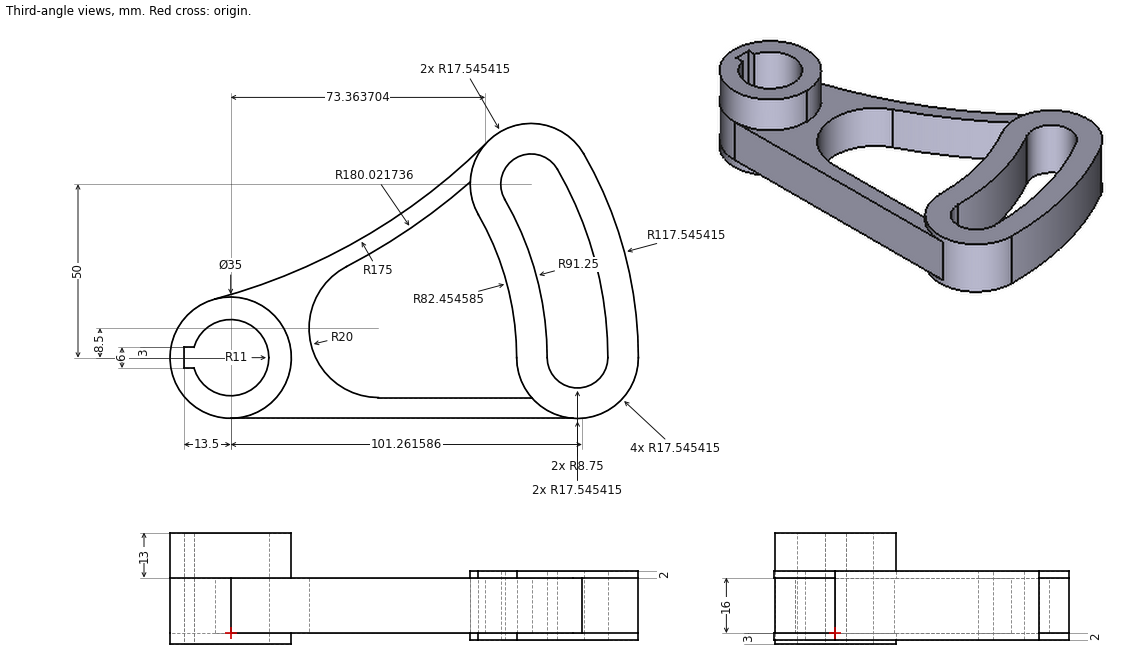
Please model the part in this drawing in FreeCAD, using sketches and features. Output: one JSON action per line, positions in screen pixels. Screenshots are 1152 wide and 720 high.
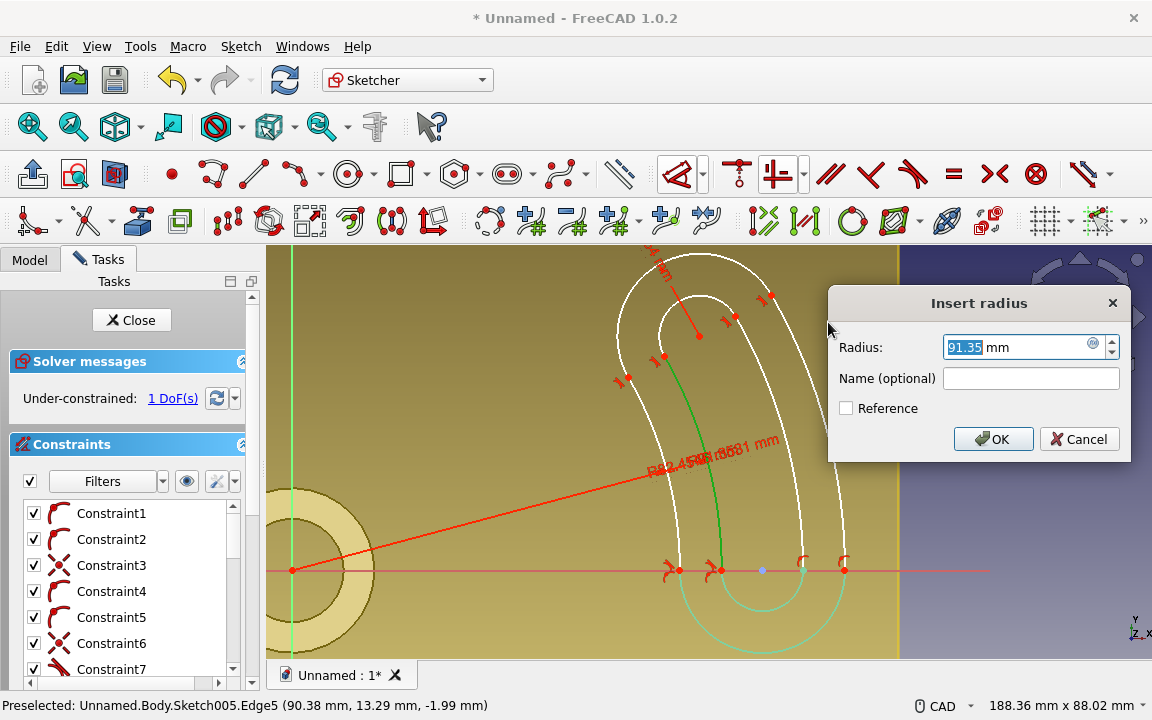
{"action": "type", "text": "91.25"}
{"action": "key", "text": "Return"}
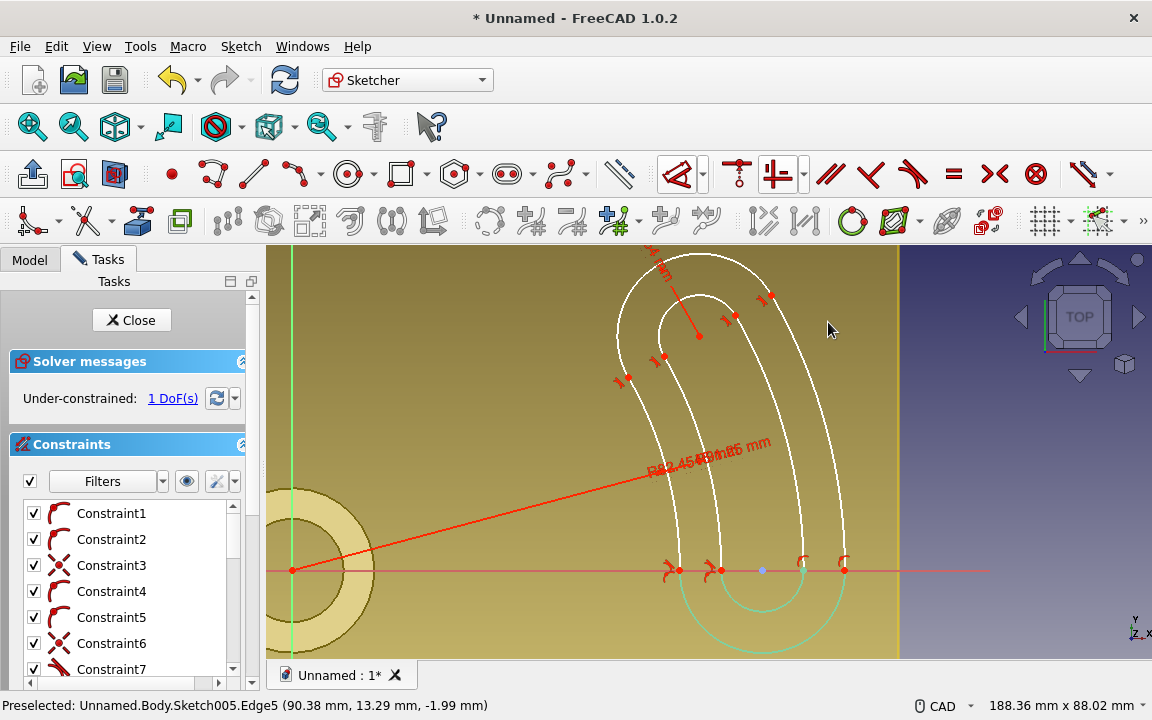
{"action": "left_click", "coordinate": [700, 336]}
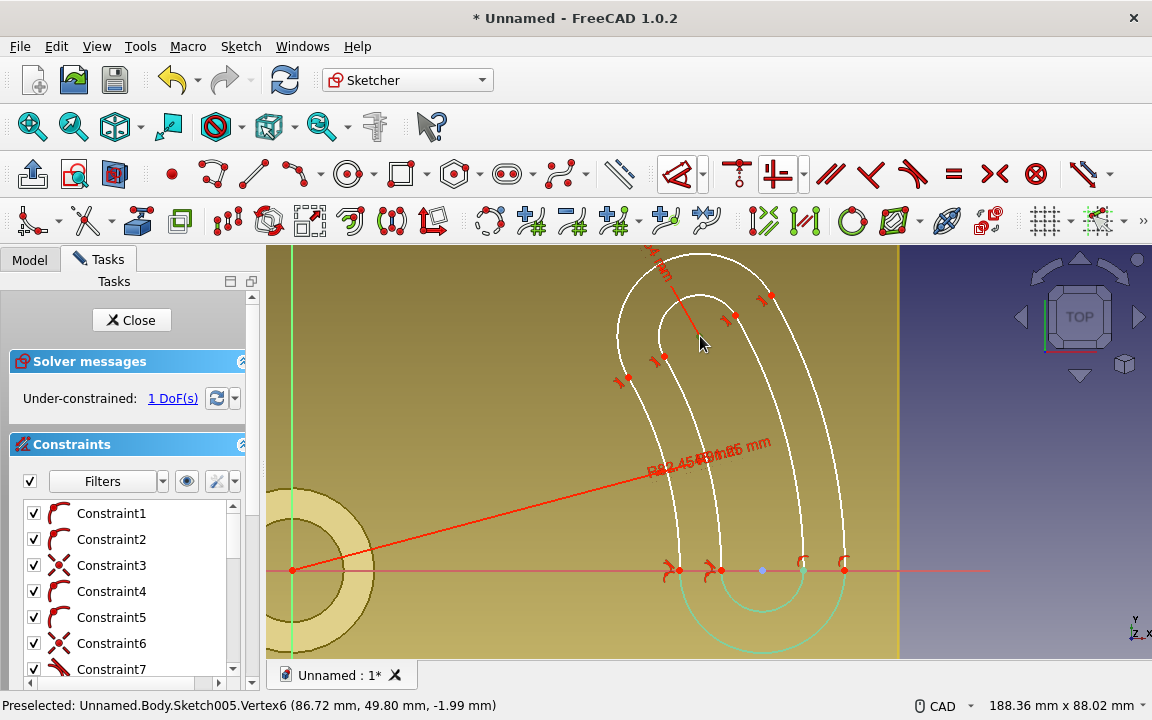
{"action": "left_click", "coordinate": [702, 174]}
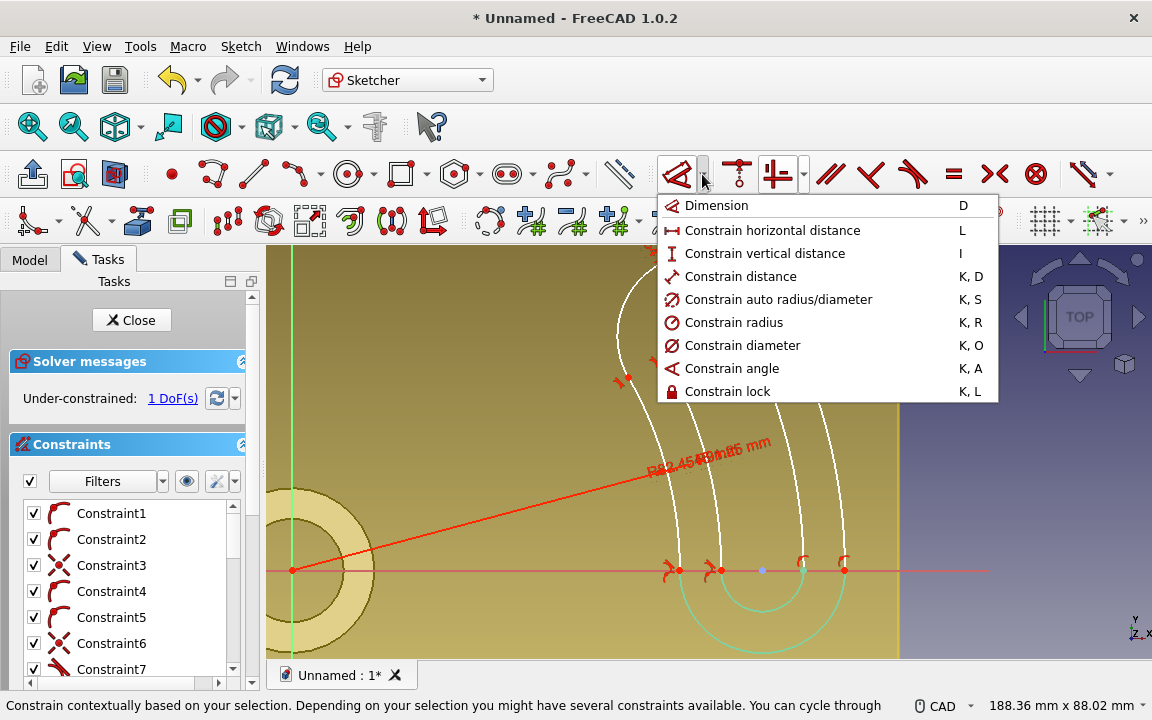
{"action": "left_click", "coordinate": [828, 254]}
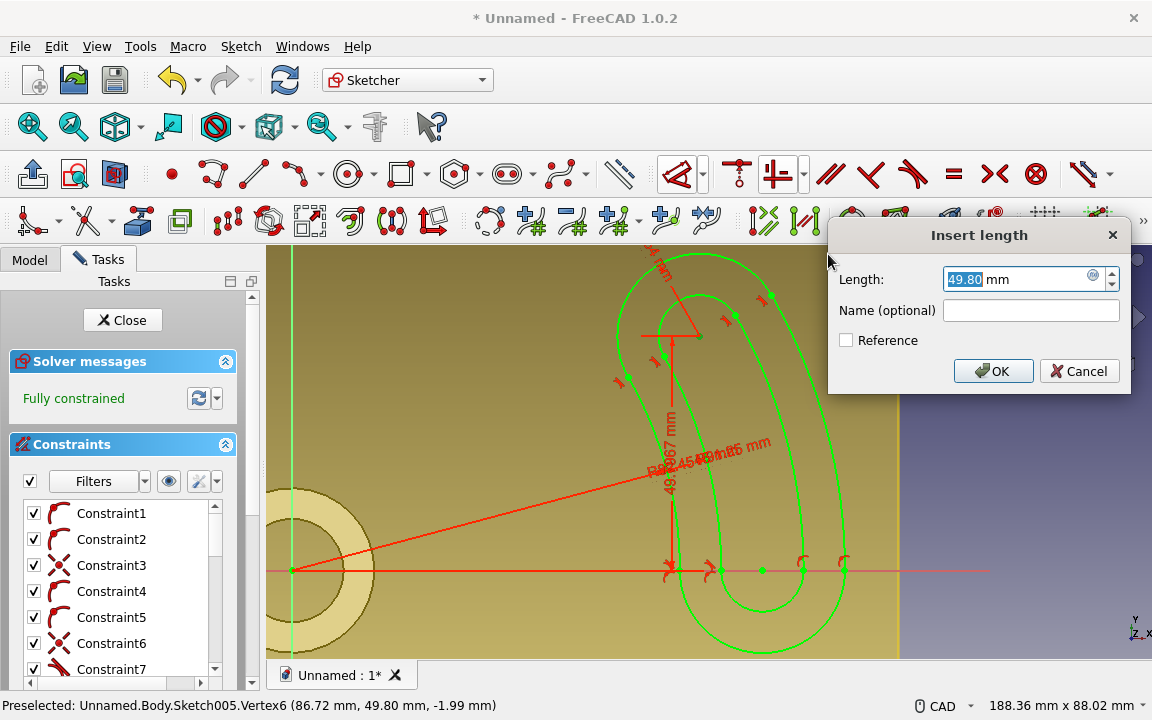
{"action": "type", "text": "50"}
{"action": "key", "text": "Return"}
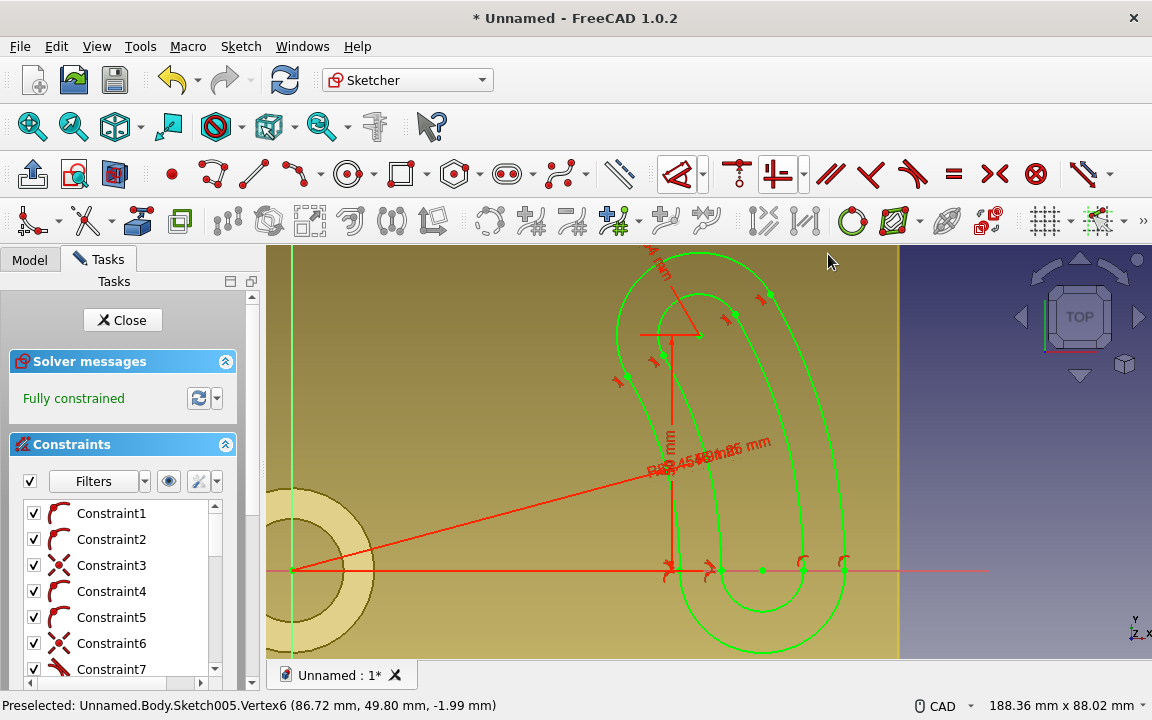
{"action": "left_click", "coordinate": [123, 320]}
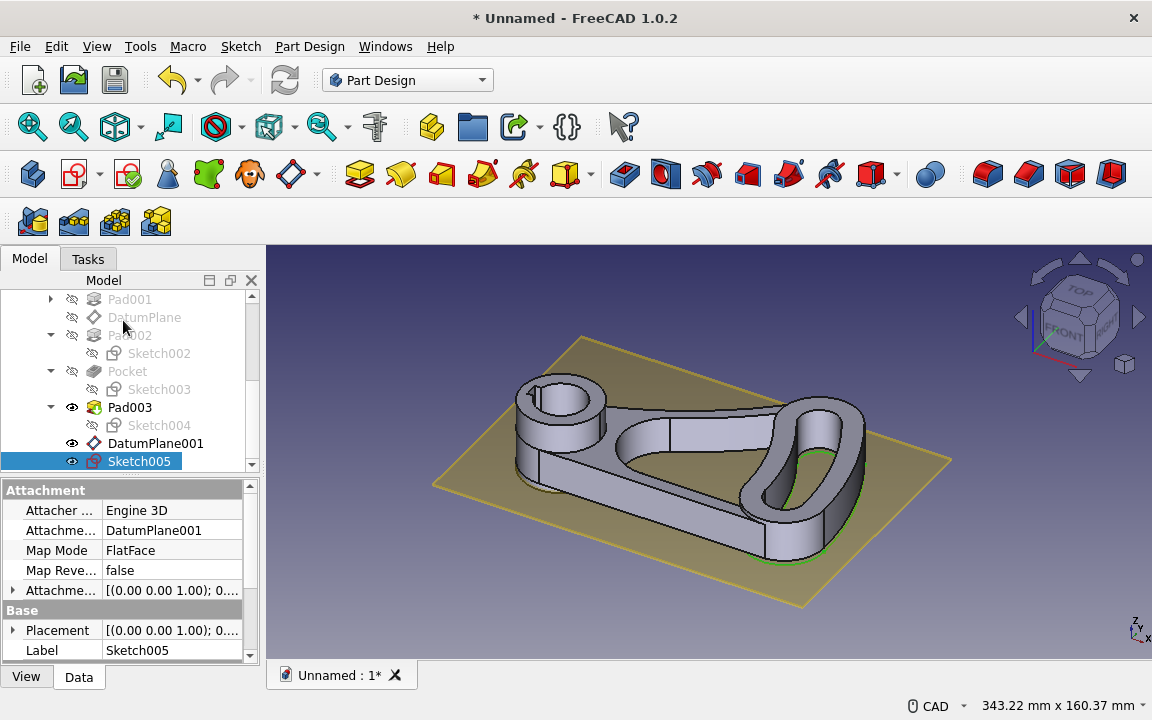
{"action": "left_click", "coordinate": [360, 174]}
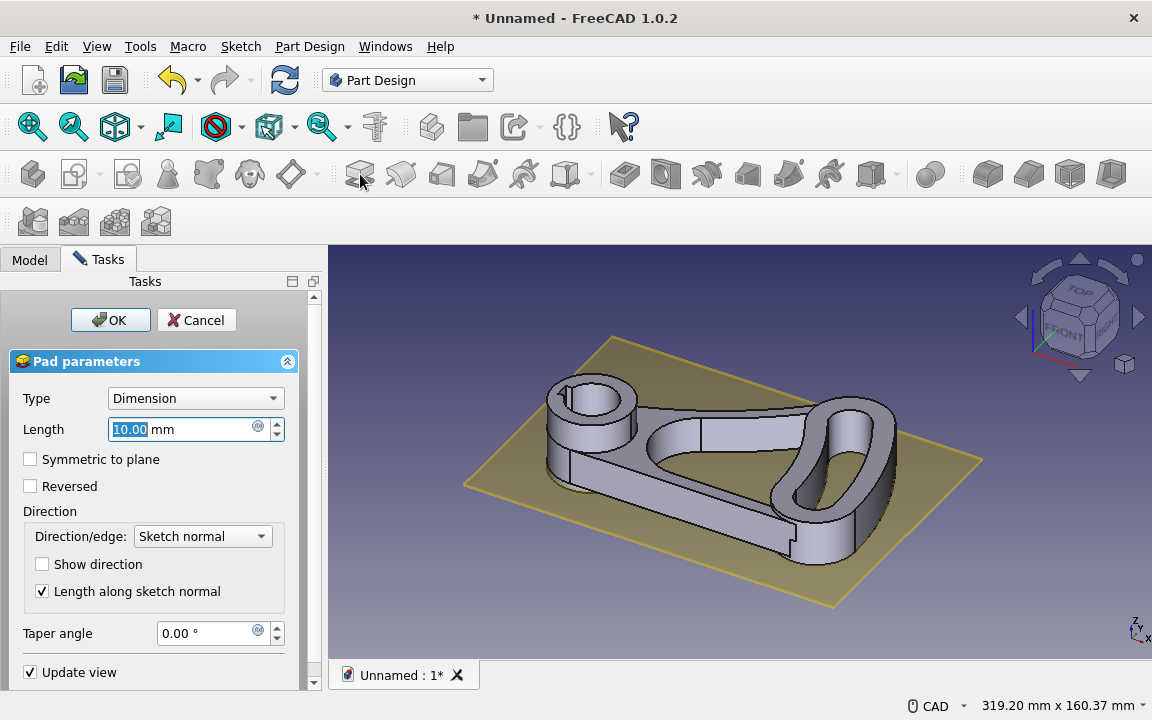
{"action": "type", "text": "2"}
{"action": "key", "text": "Tab"}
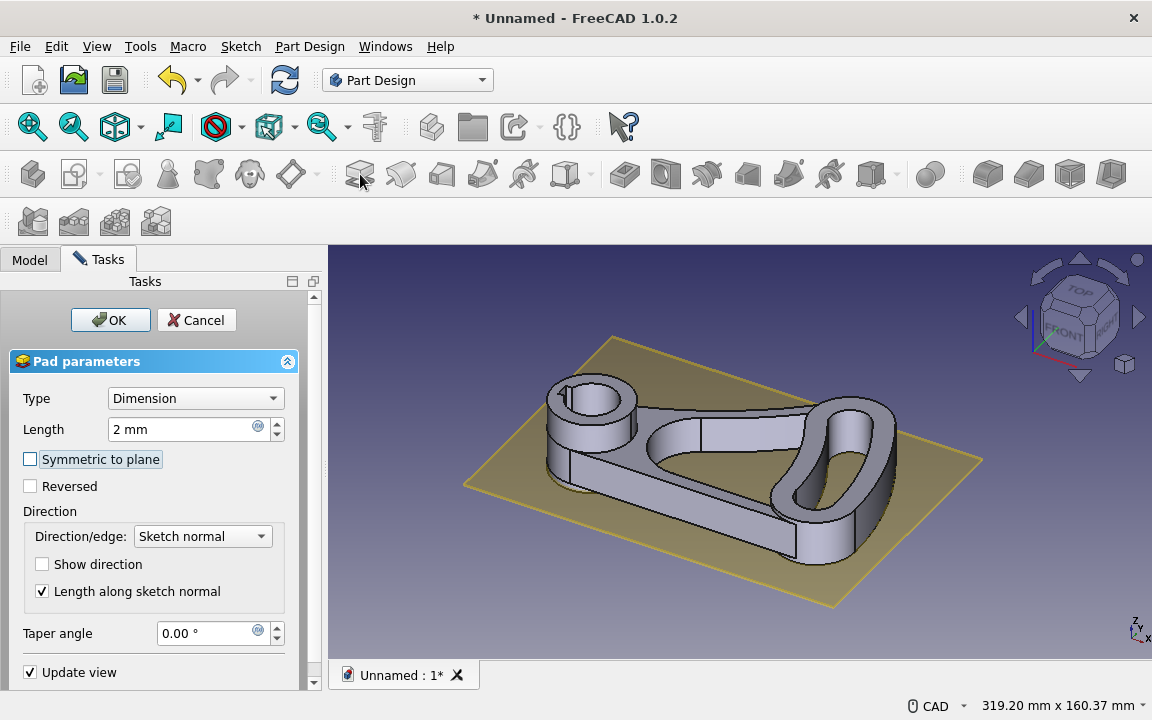
{"action": "left_click", "coordinate": [111, 320]}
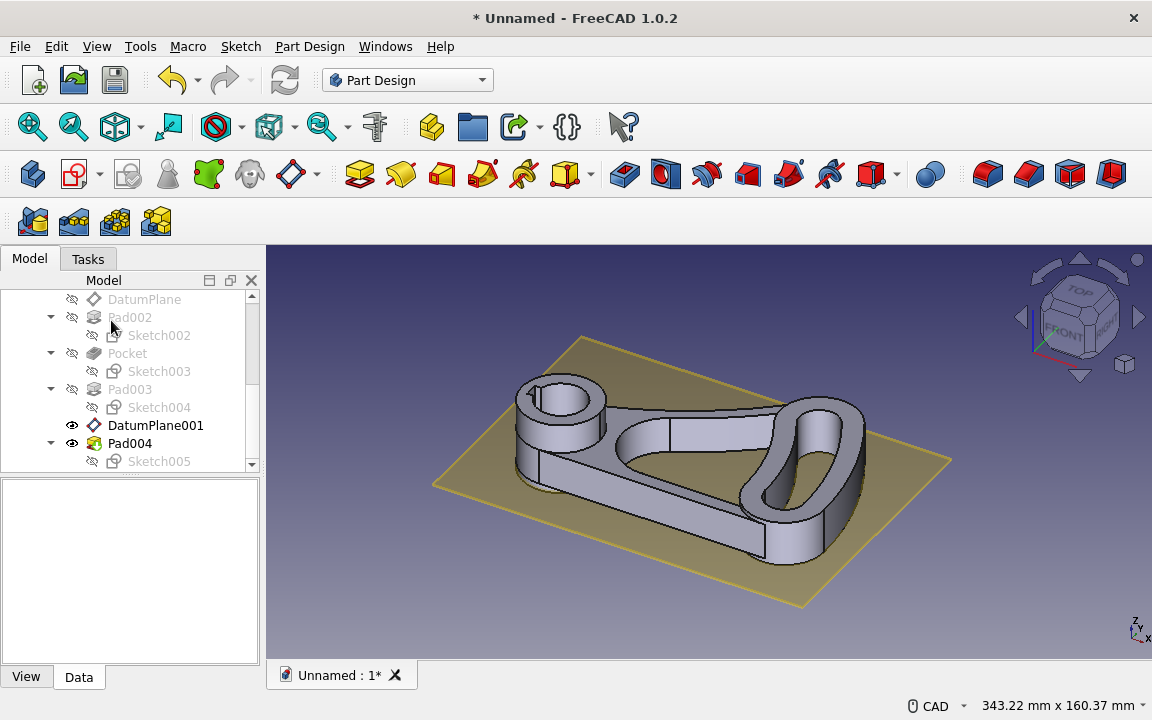
{"action": "left_click", "coordinate": [117, 425]}
{"action": "key", "text": "space"}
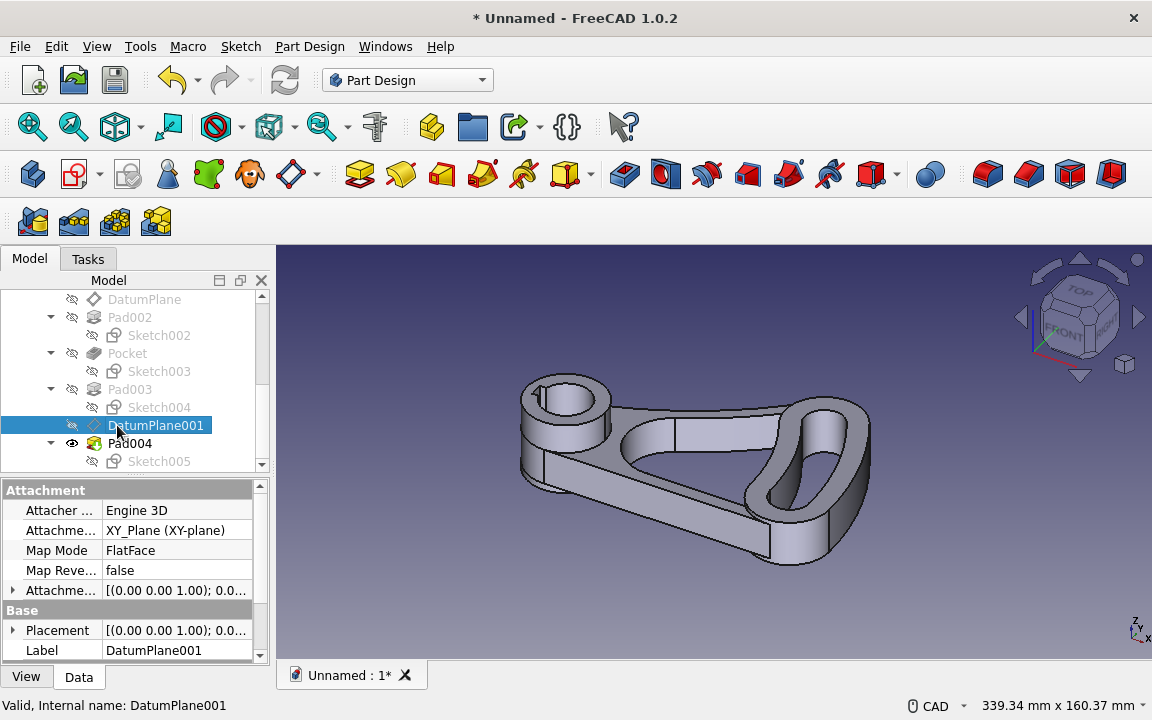
{"action": "key", "text": "0"}